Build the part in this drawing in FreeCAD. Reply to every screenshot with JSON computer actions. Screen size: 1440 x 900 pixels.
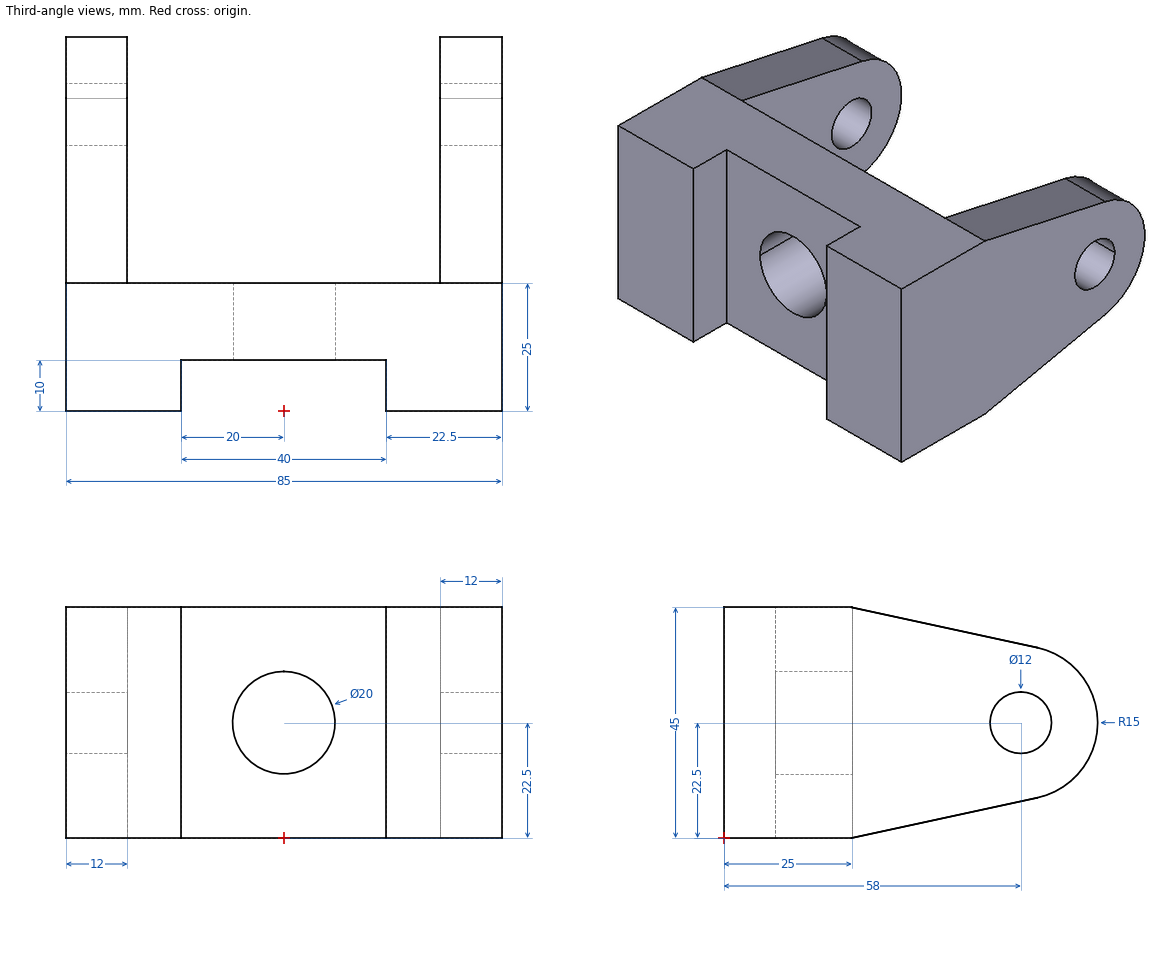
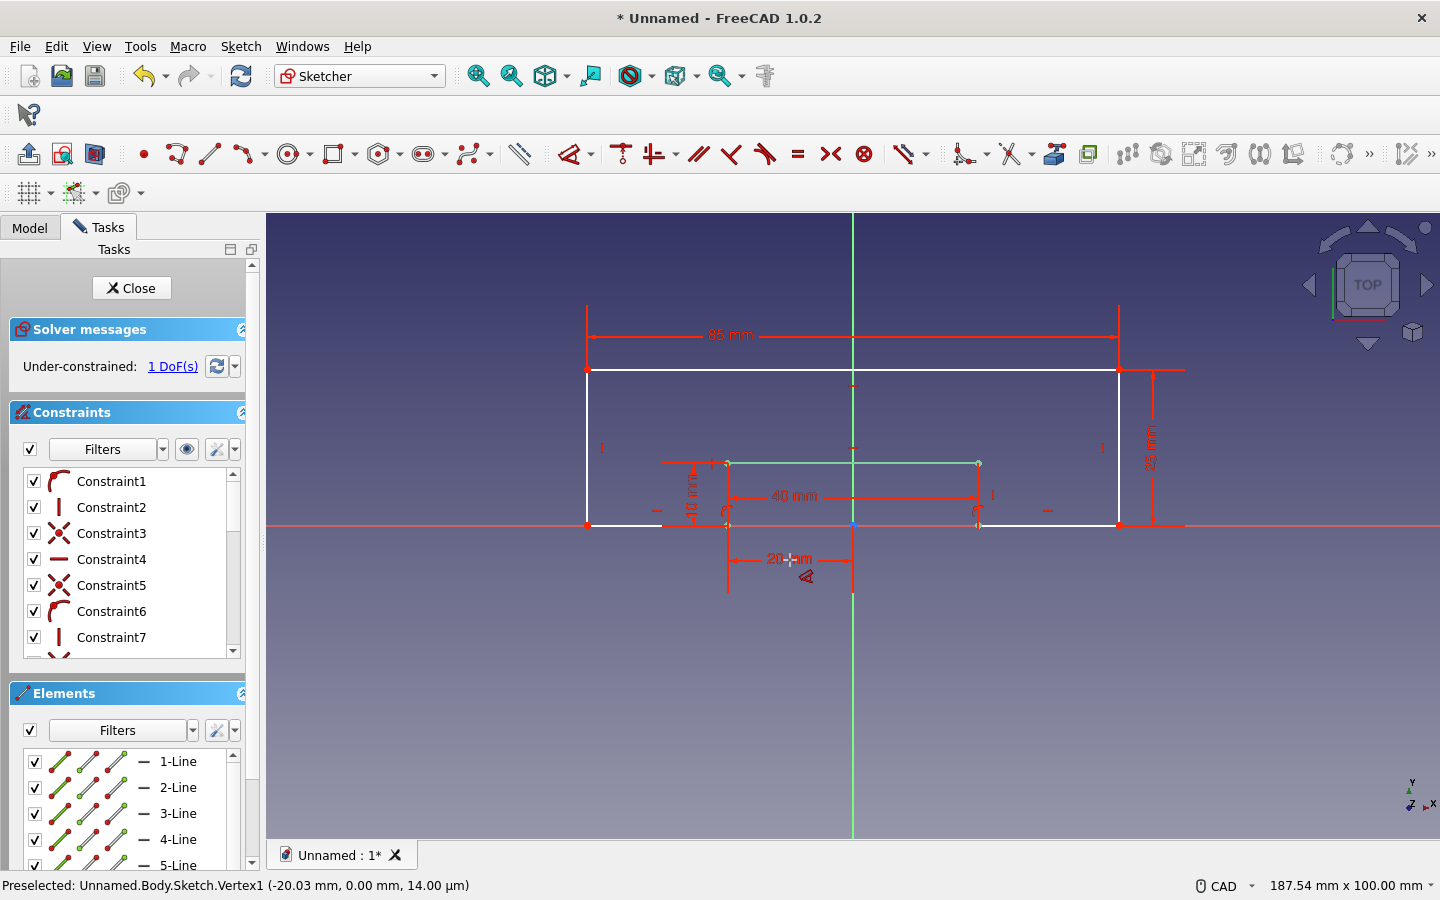
{"action": "left_click", "coordinate": [1020, 526]}
{"action": "left_click", "coordinate": [1049, 560]}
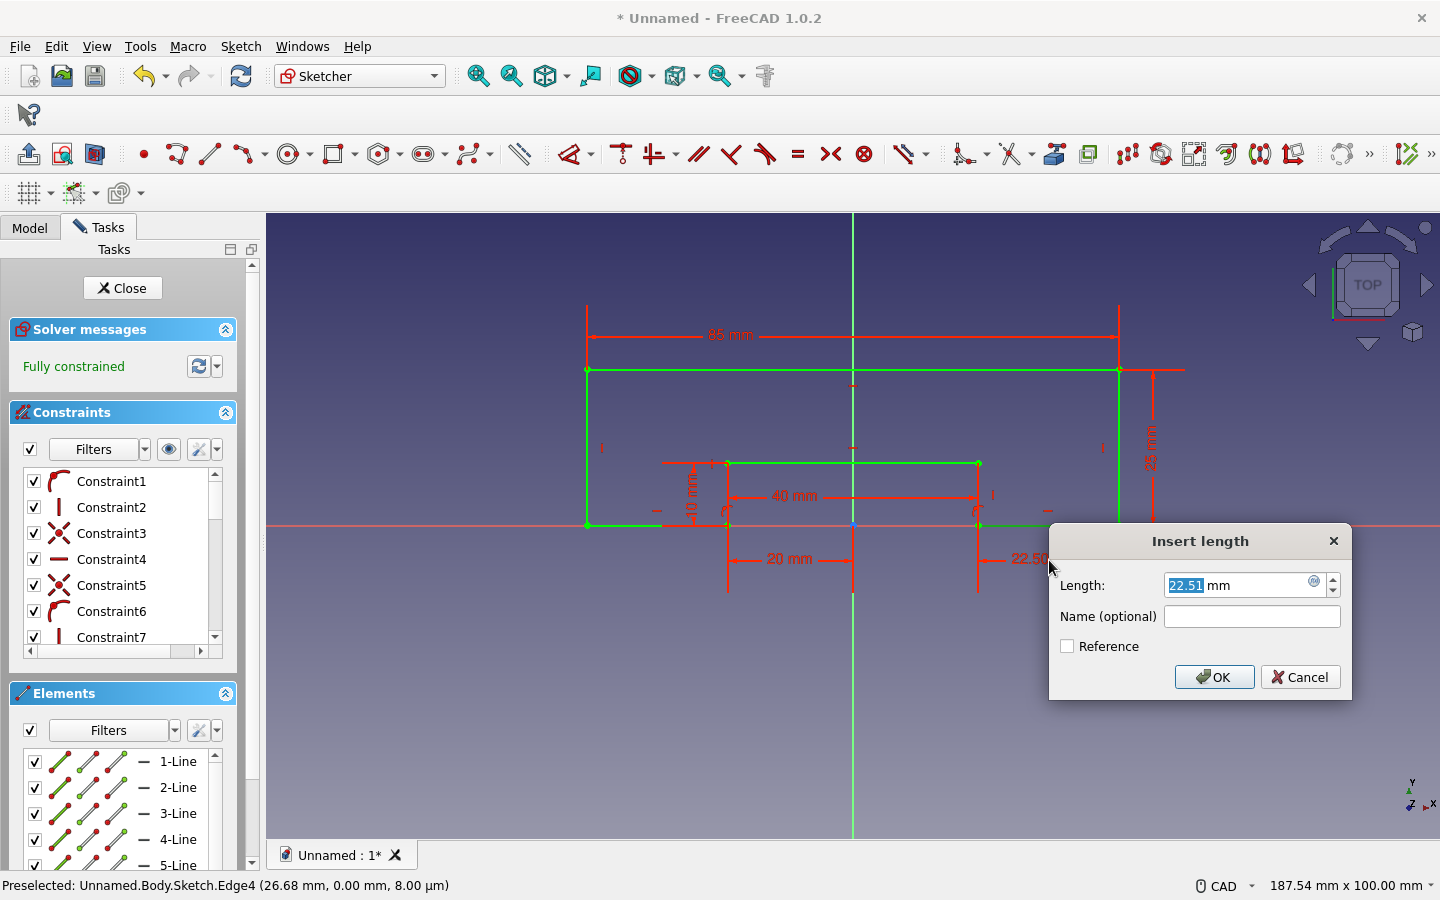
{"action": "type", "text": "22.5"}
{"action": "key", "text": "Return"}
{"action": "key", "text": "Escape"}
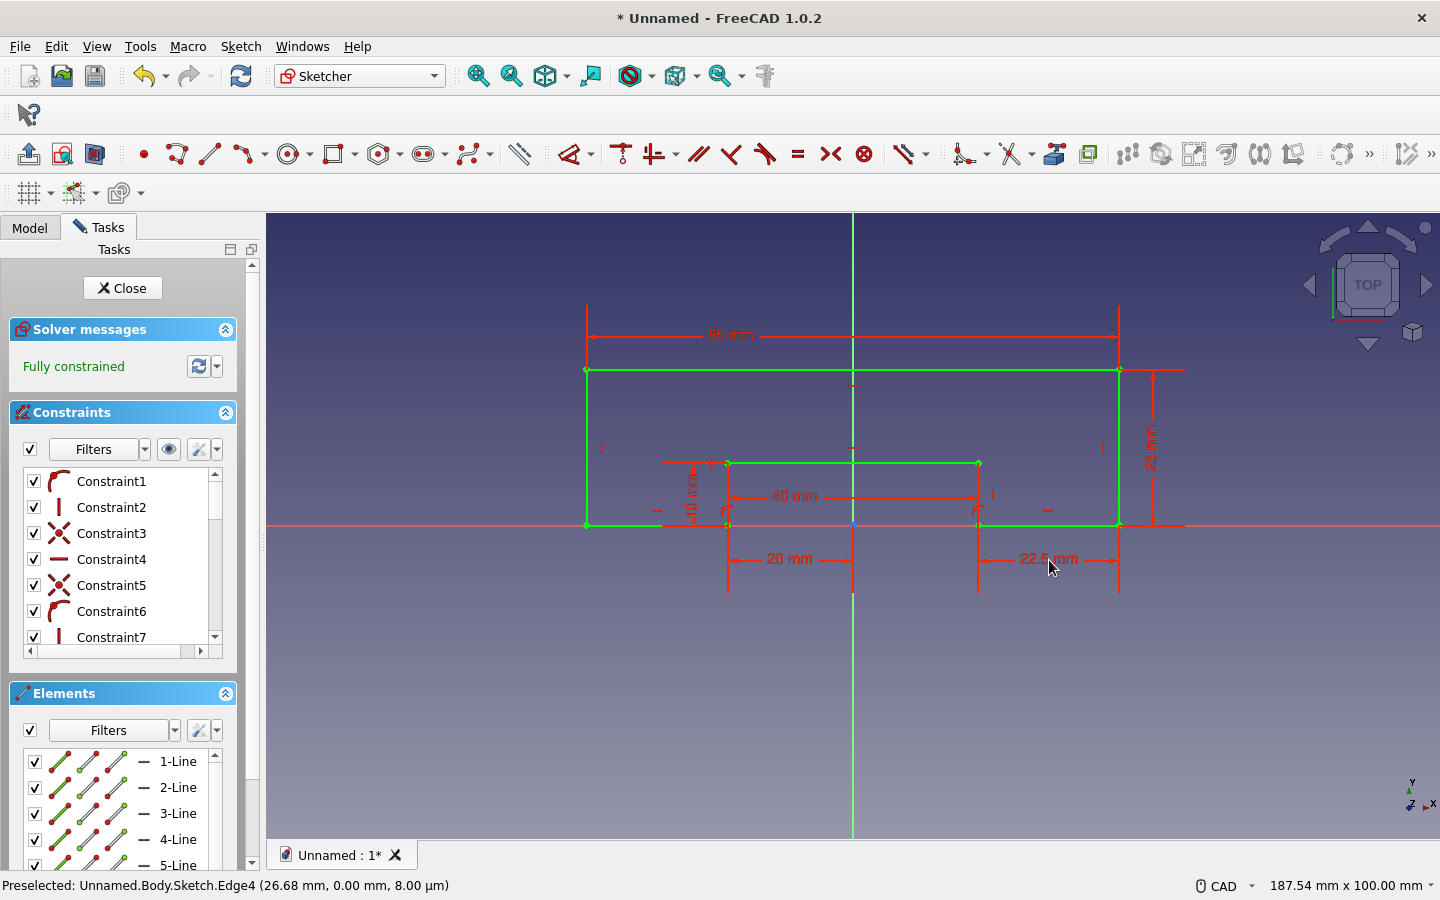
{"action": "left_click", "coordinate": [123, 288]}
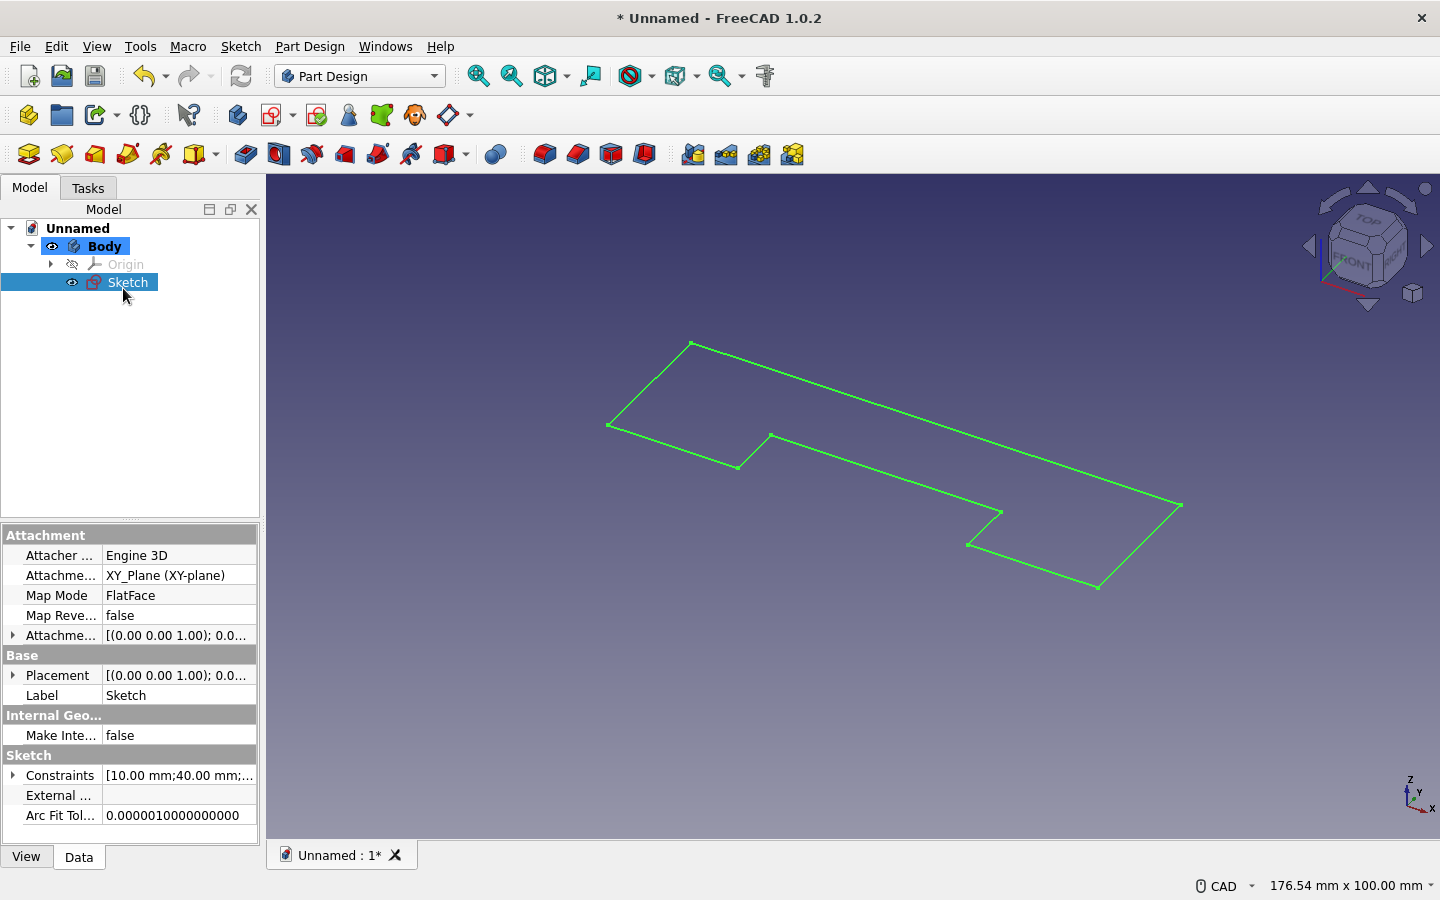
{"action": "left_click", "coordinate": [29, 154]}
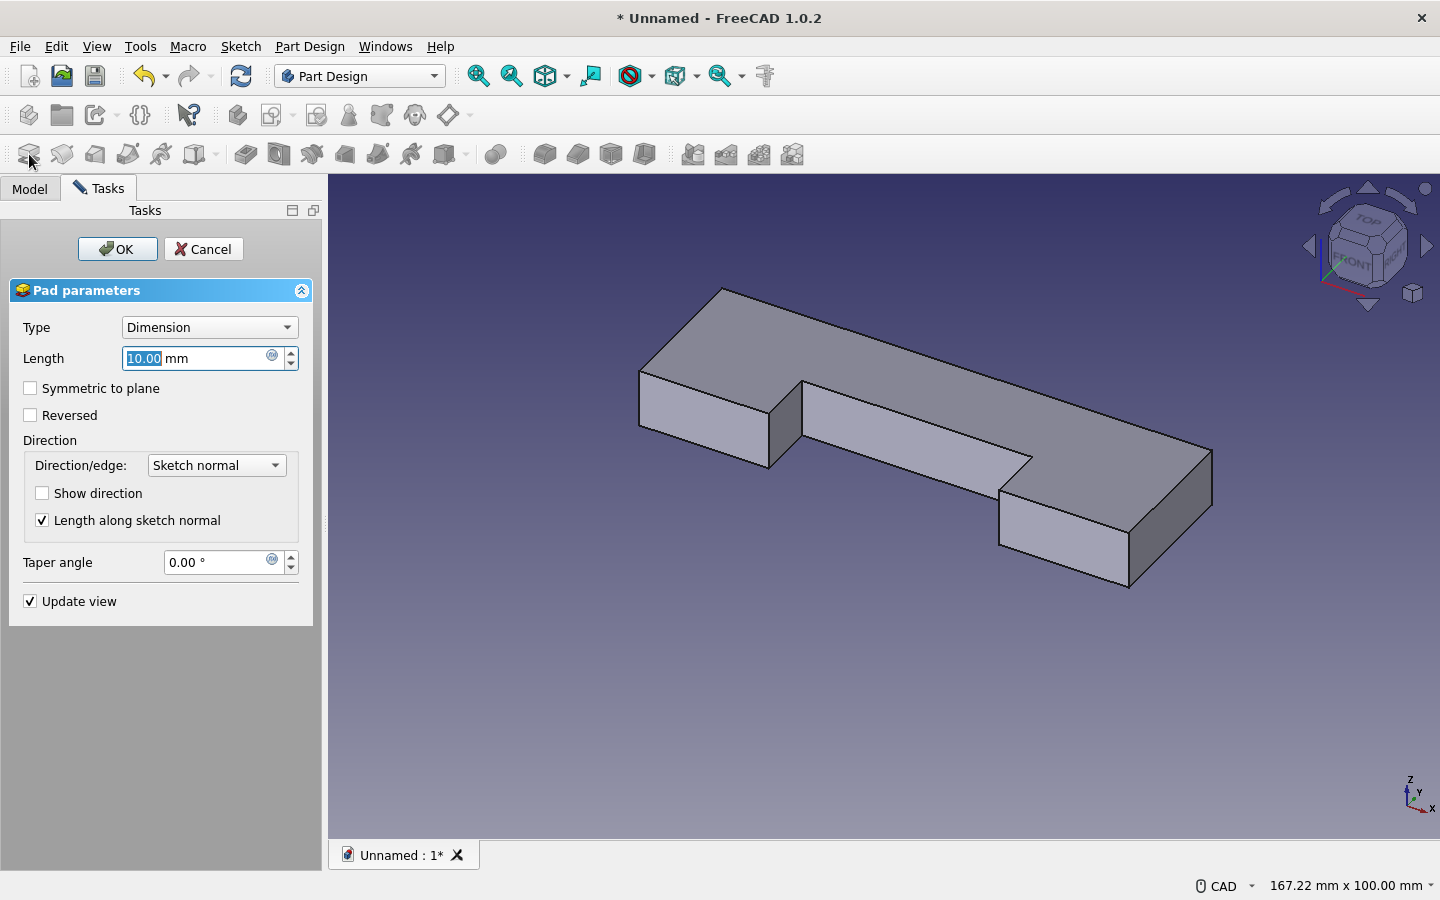
{"action": "type", "text": "45"}
{"action": "key", "text": "Tab"}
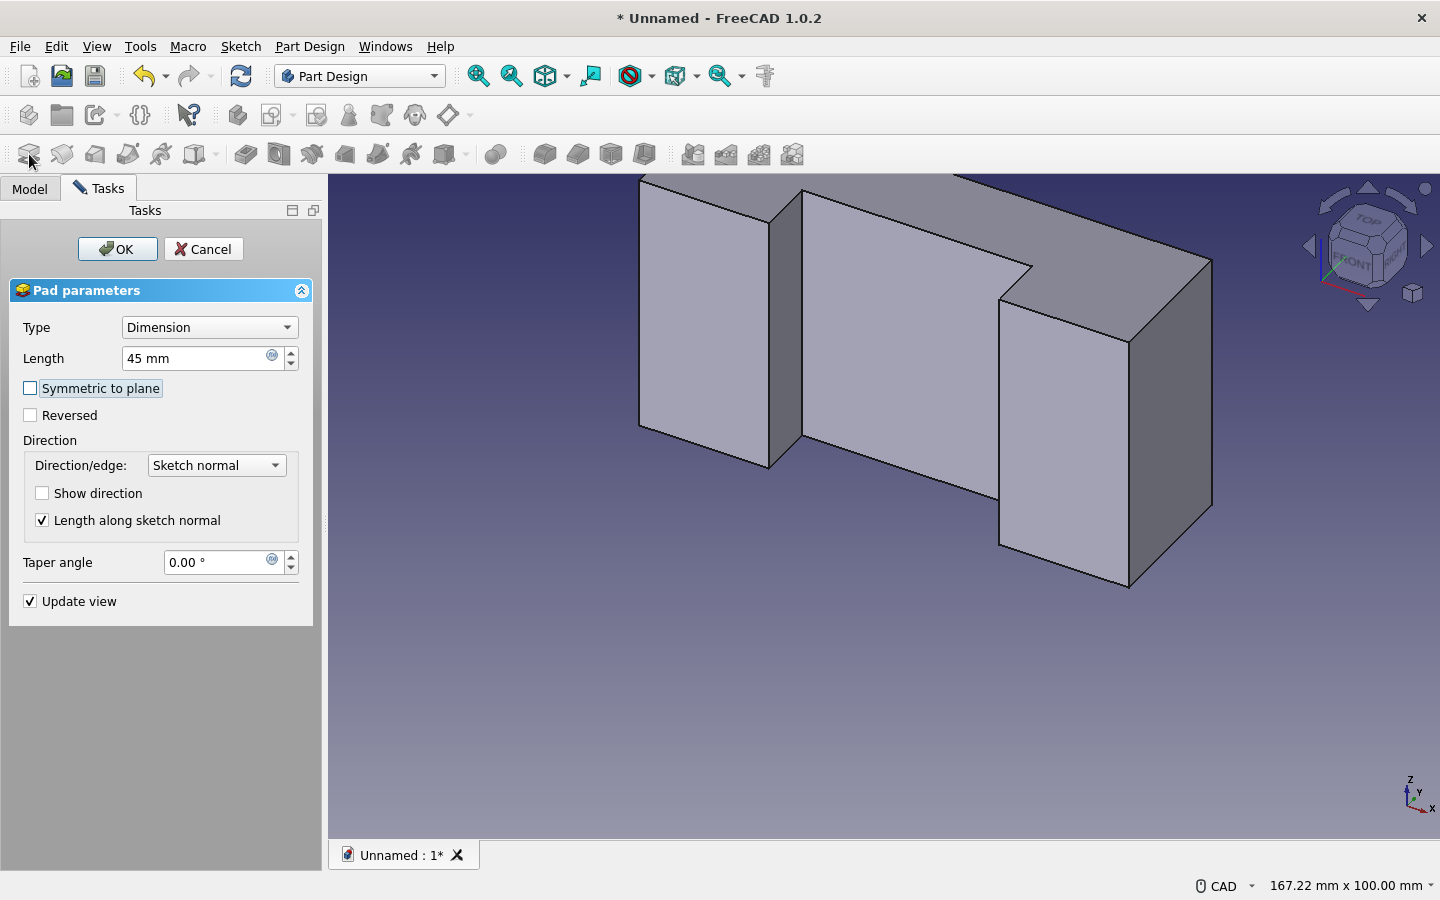
{"action": "left_click", "coordinate": [118, 249]}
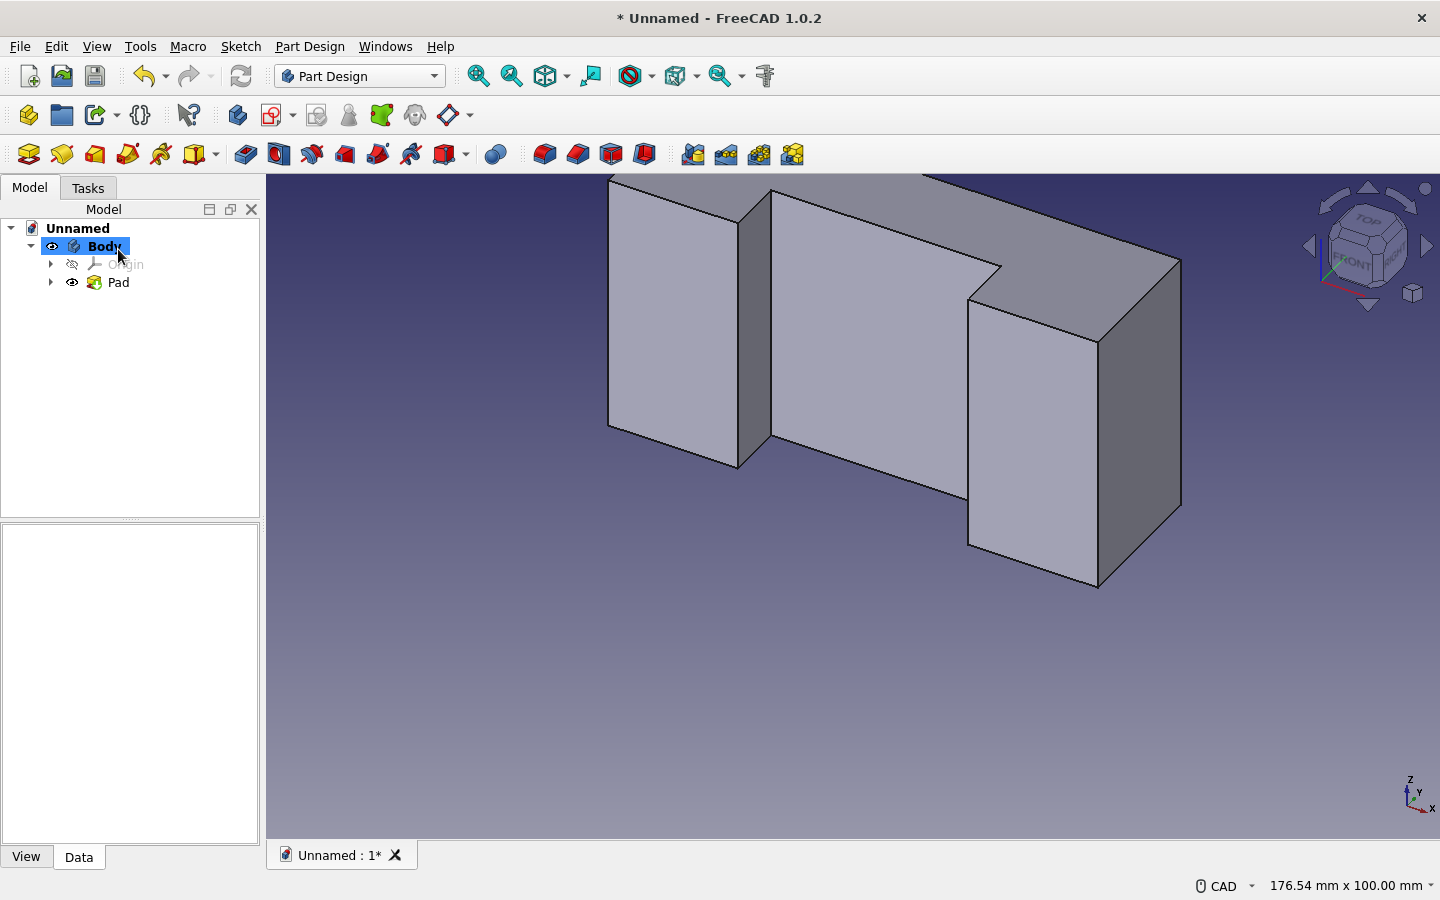
{"action": "left_click", "coordinate": [479, 76]}